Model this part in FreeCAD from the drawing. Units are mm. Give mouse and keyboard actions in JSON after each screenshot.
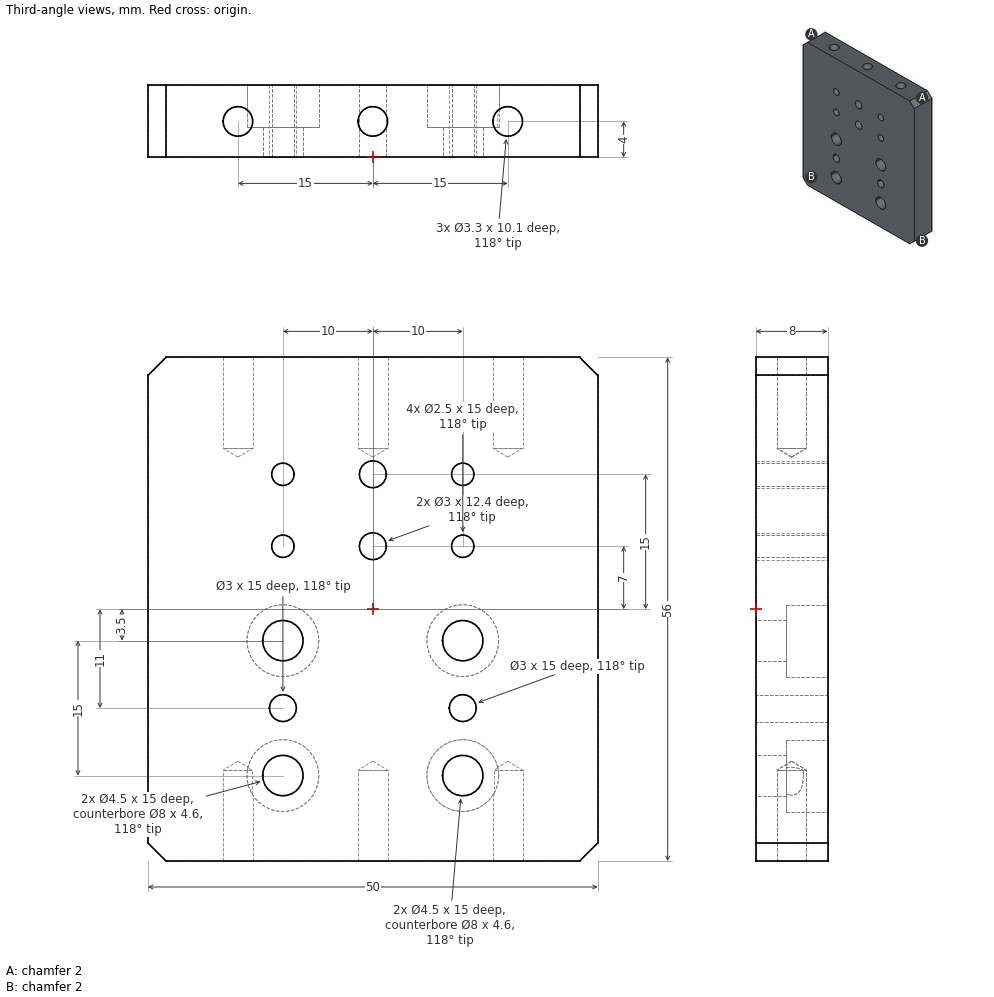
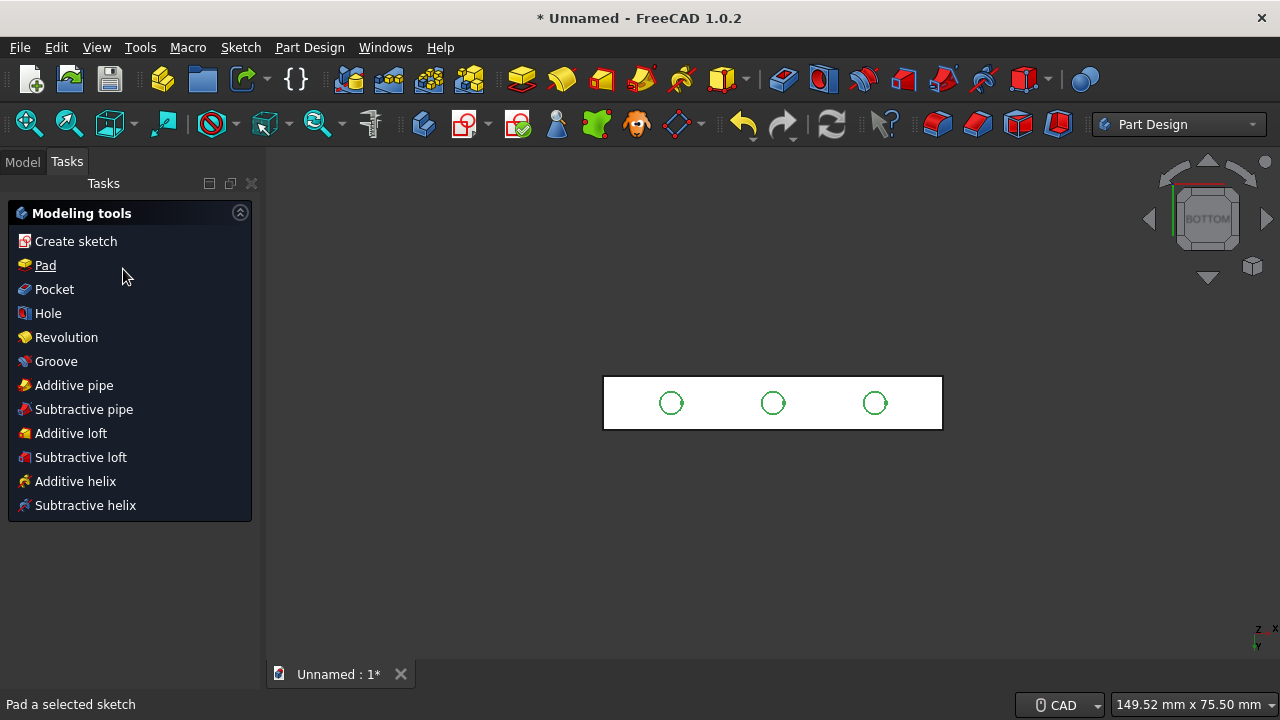
{"action": "left_click", "coordinate": [824, 80]}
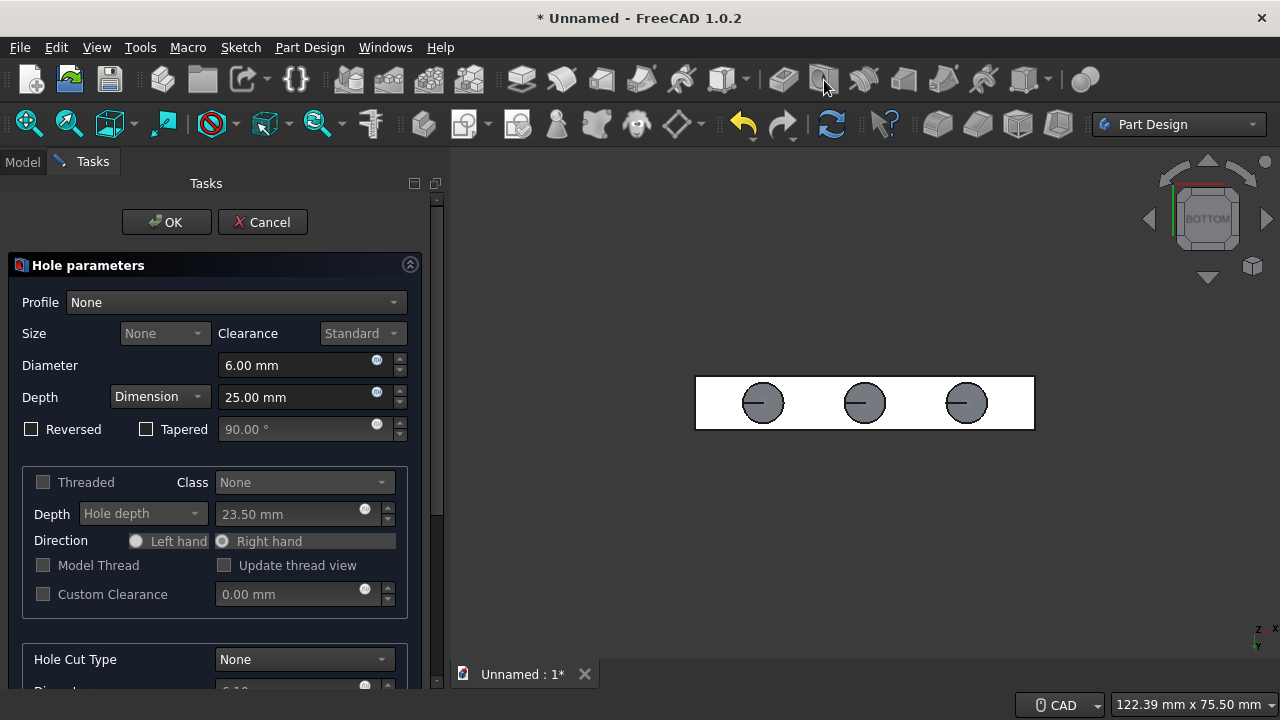
{"action": "triple_click", "coordinate": [305, 365]}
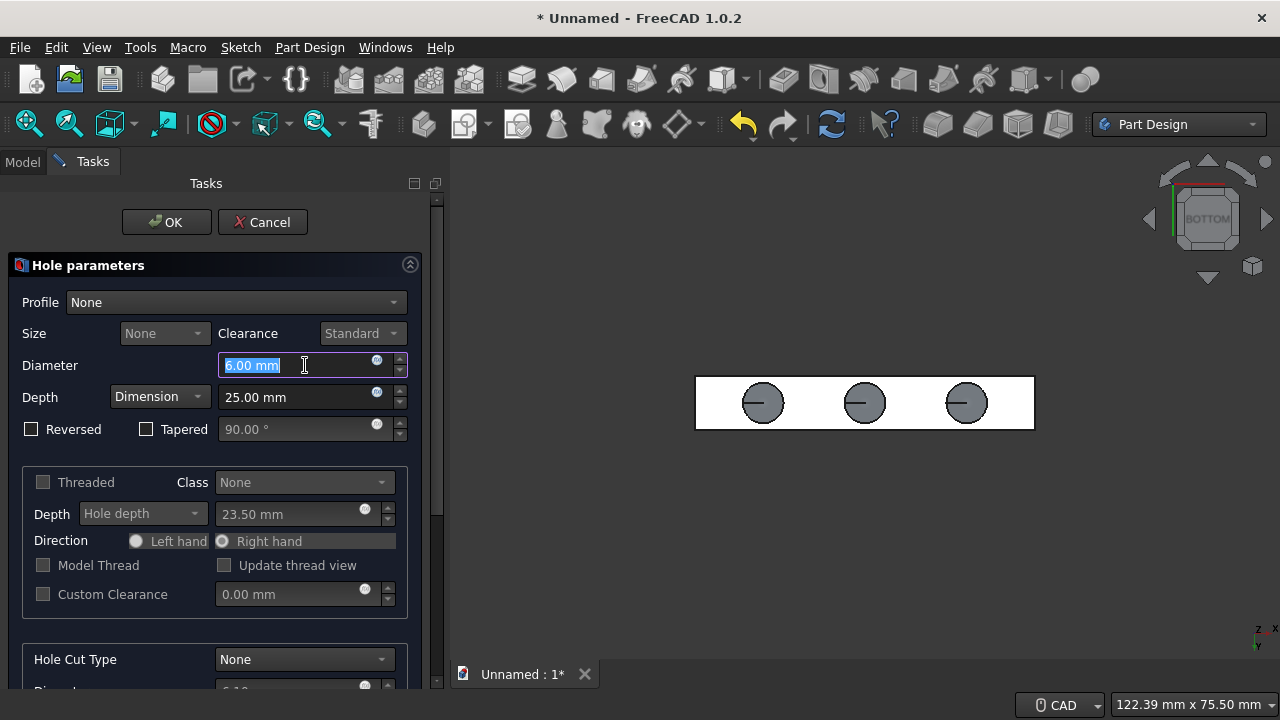
{"action": "type", "text": "3.3"}
{"action": "key", "text": "Tab"}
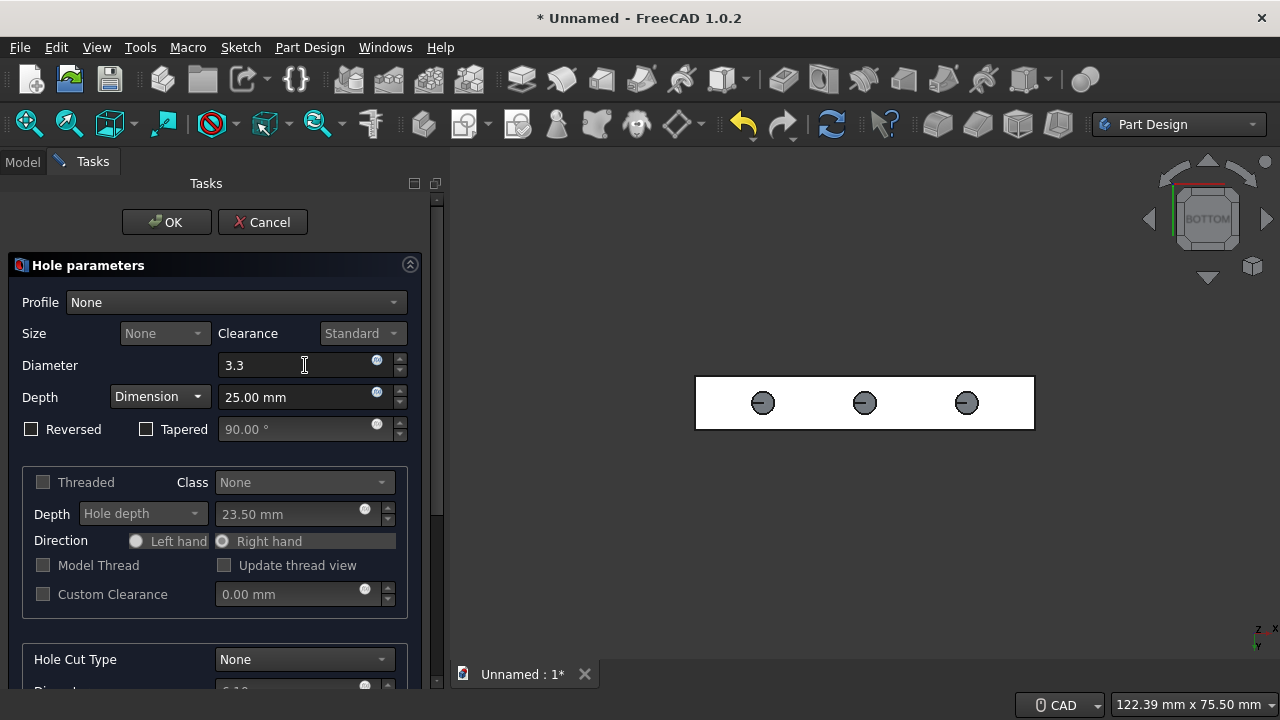
{"action": "triple_click", "coordinate": [305, 397]}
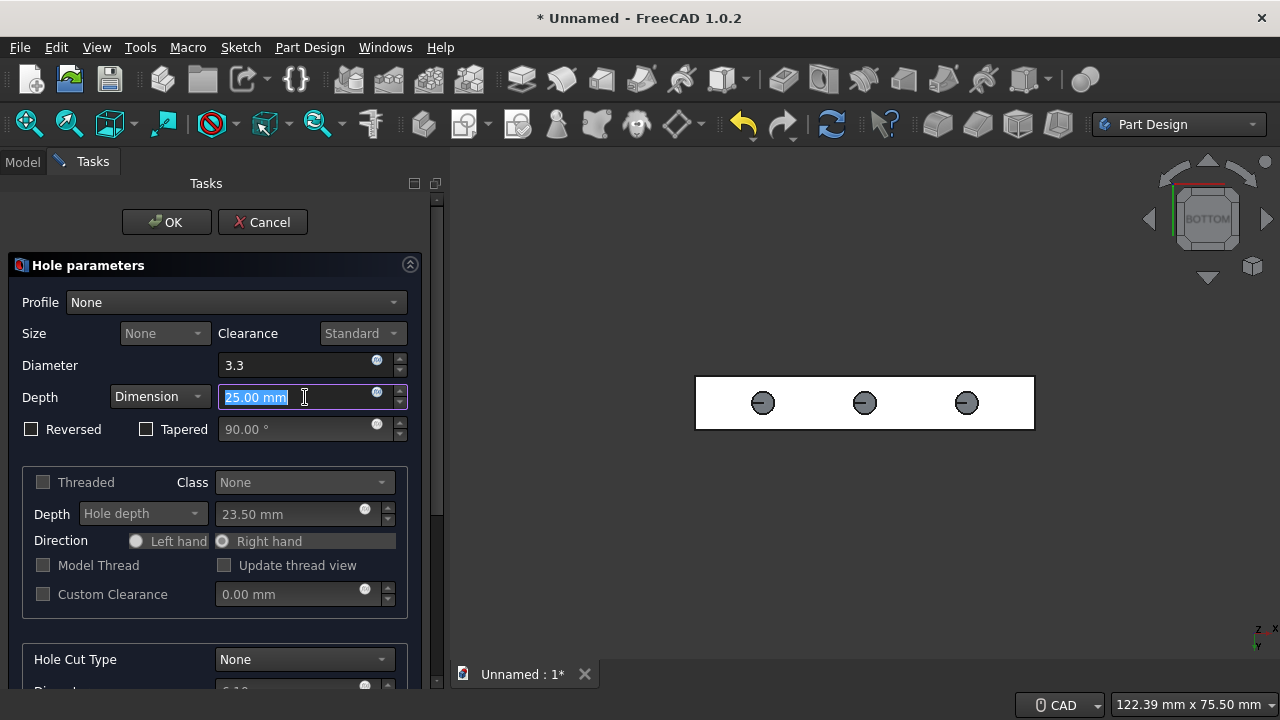
{"action": "type", "text": "10.1"}
{"action": "key", "text": "Tab"}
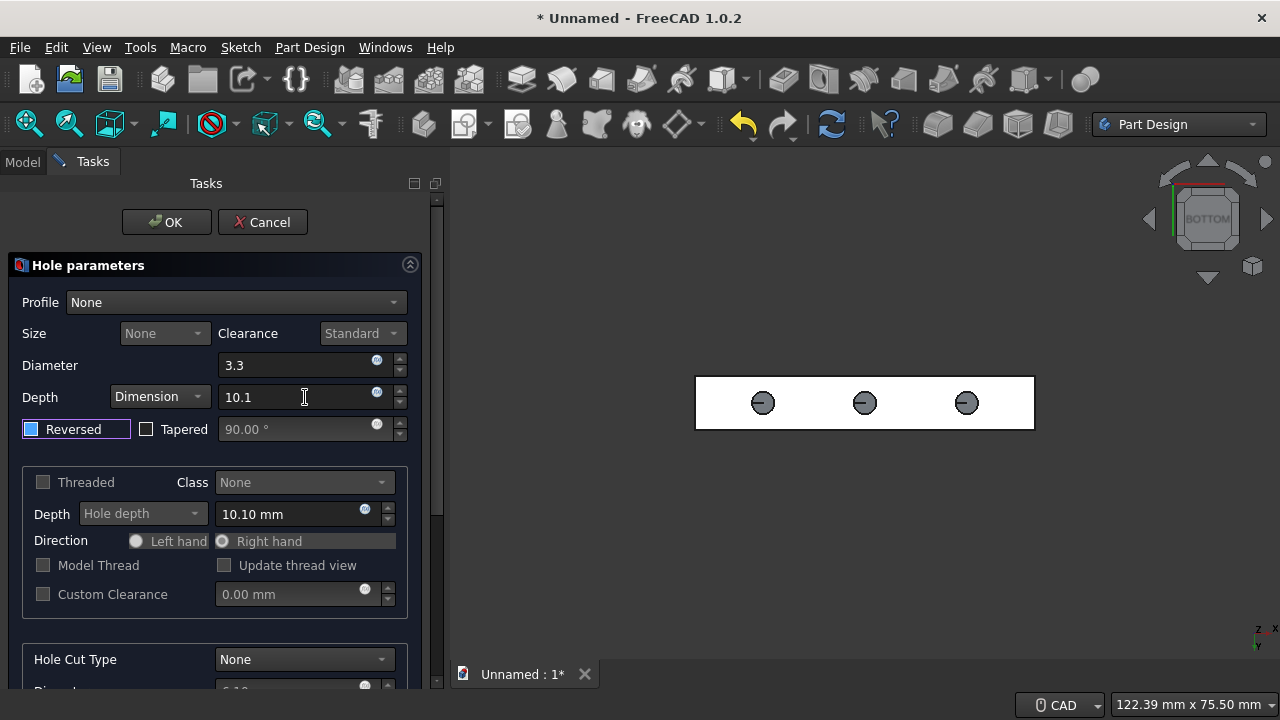
{"action": "left_click", "coordinate": [167, 222]}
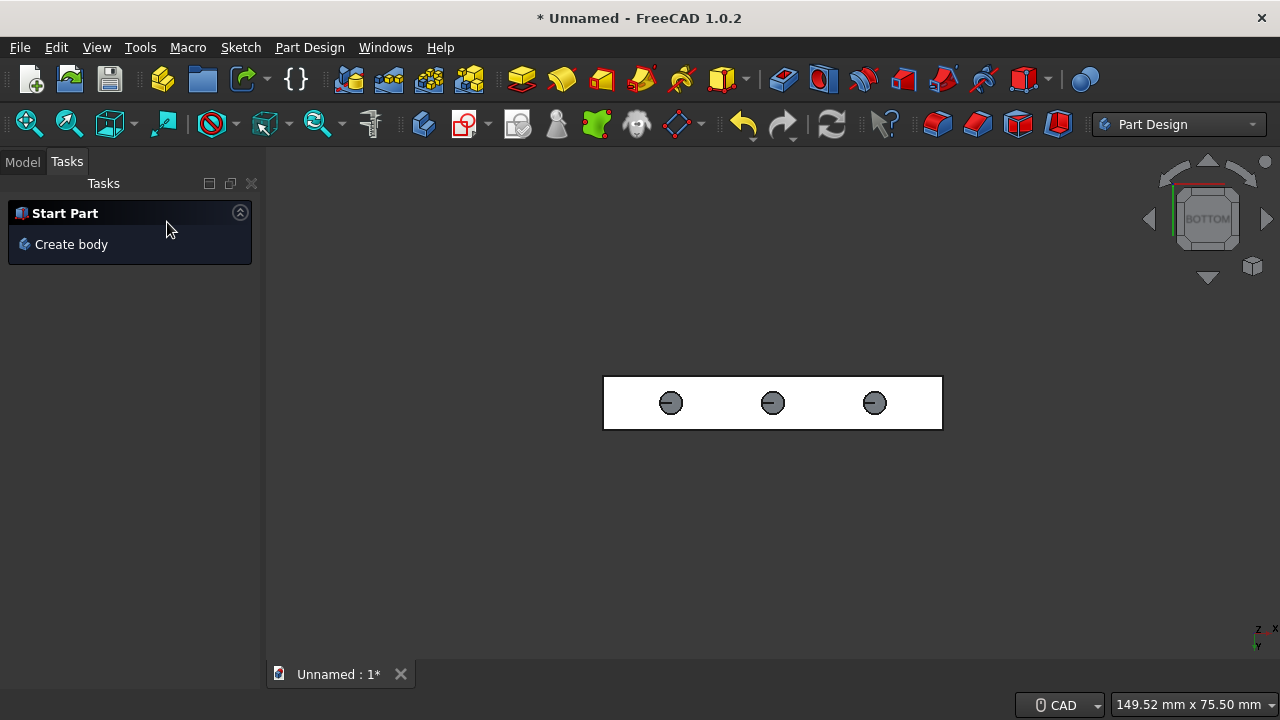
{"action": "left_click", "coordinate": [30, 124]}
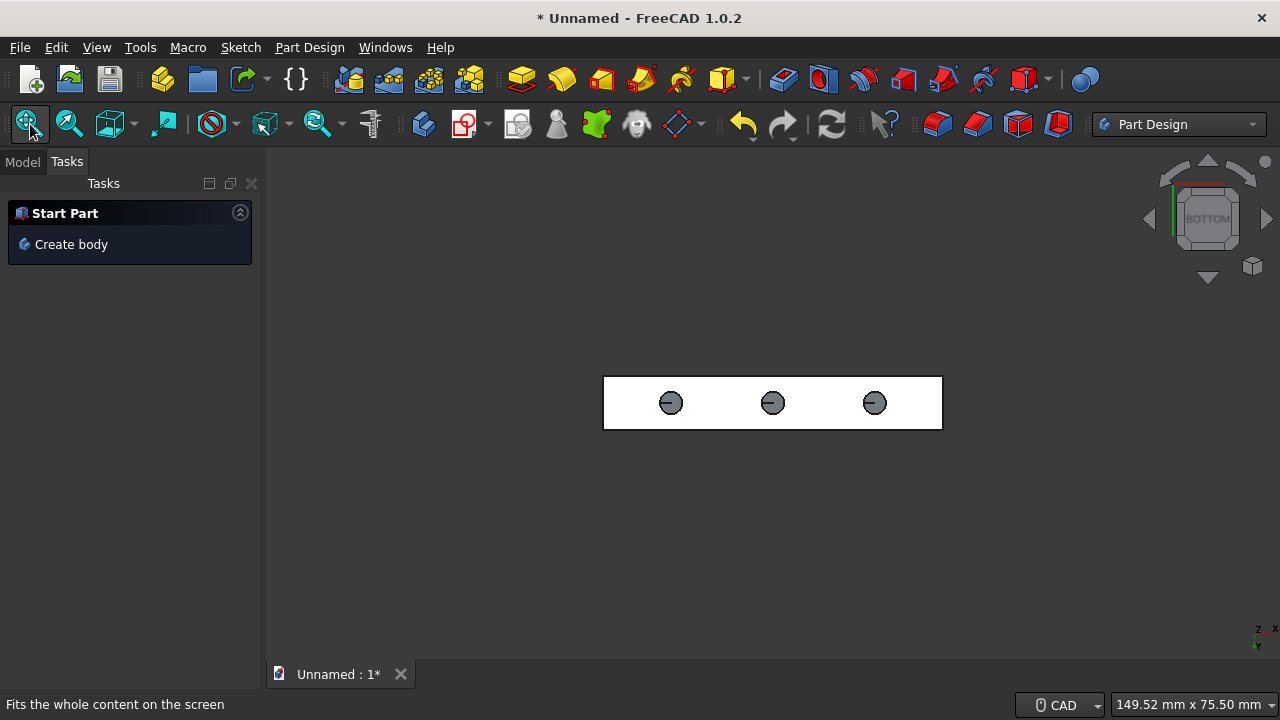
{"action": "key", "text": "0"}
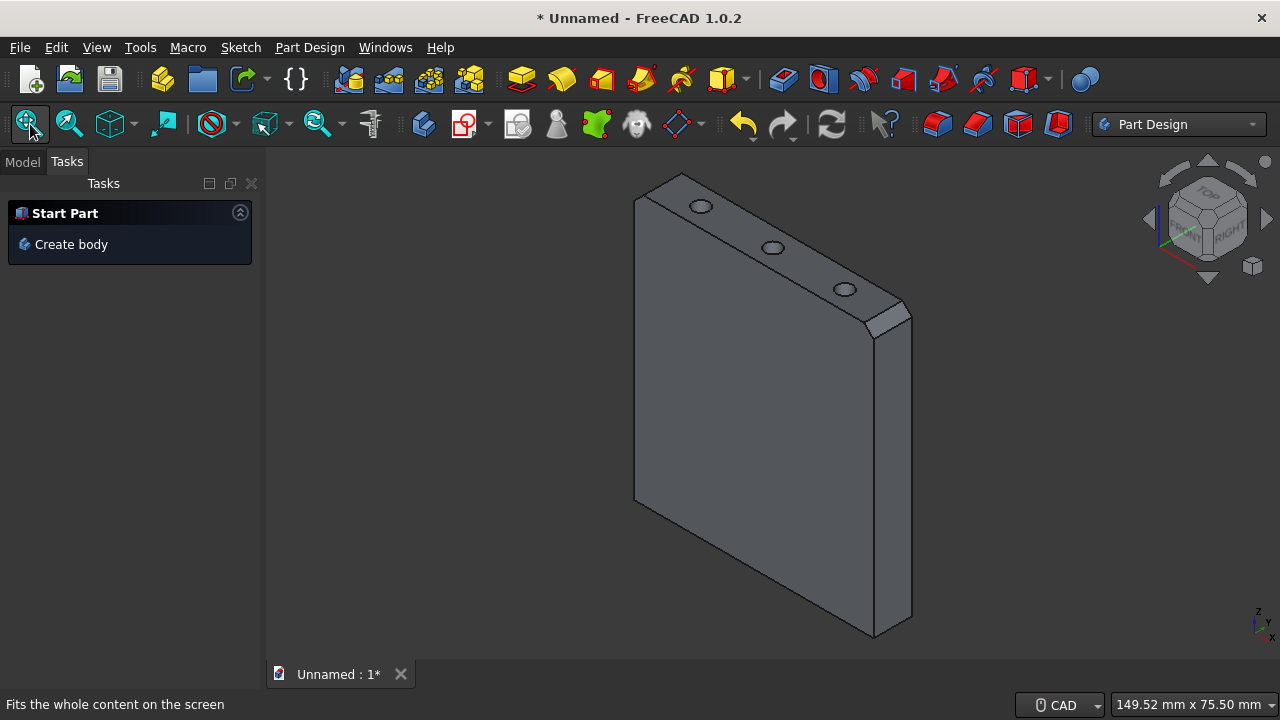
{"action": "left_click", "coordinate": [754, 413]}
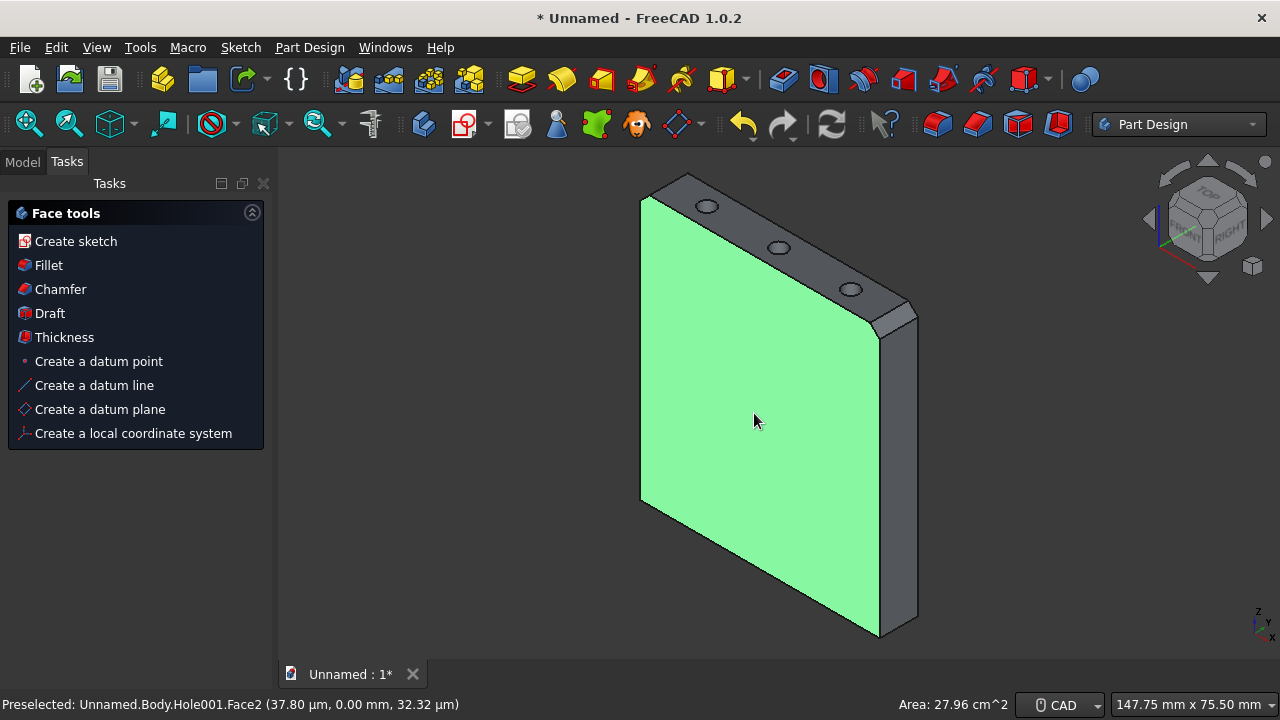
{"action": "left_click", "coordinate": [464, 124]}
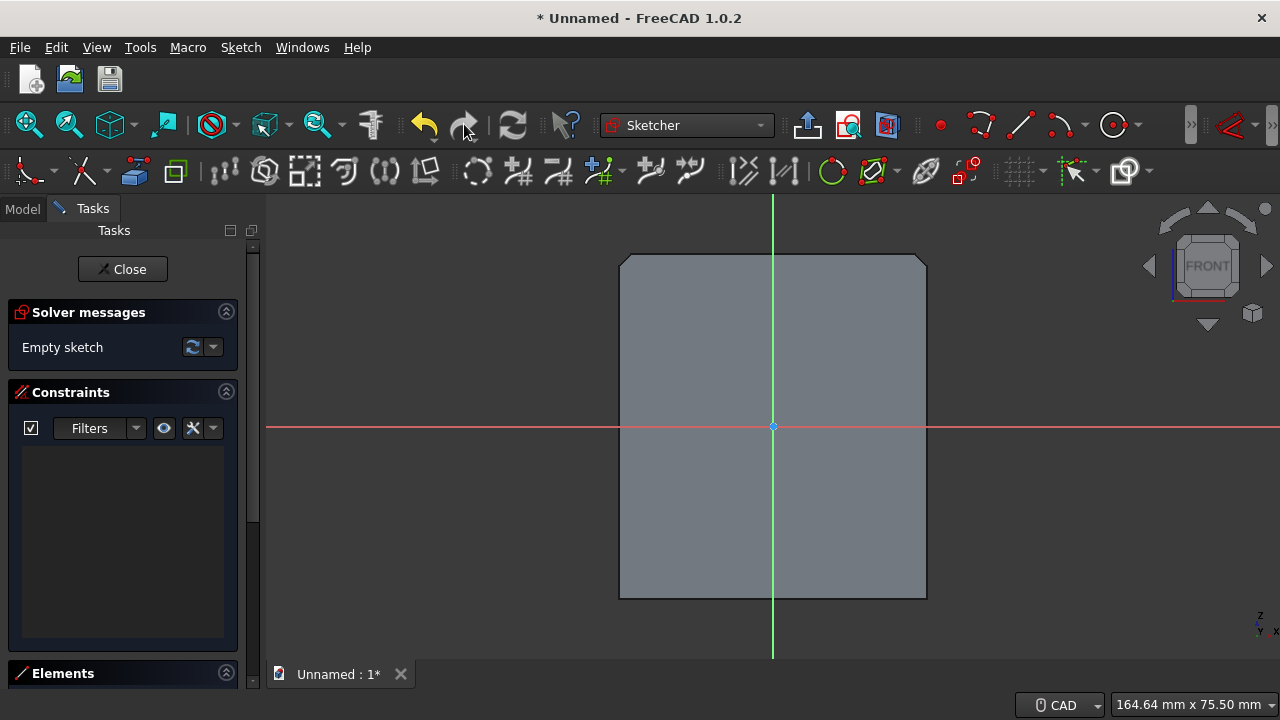
{"action": "scroll", "coordinate": [813, 346], "scroll_direction": "up", "scroll_amount": 5}